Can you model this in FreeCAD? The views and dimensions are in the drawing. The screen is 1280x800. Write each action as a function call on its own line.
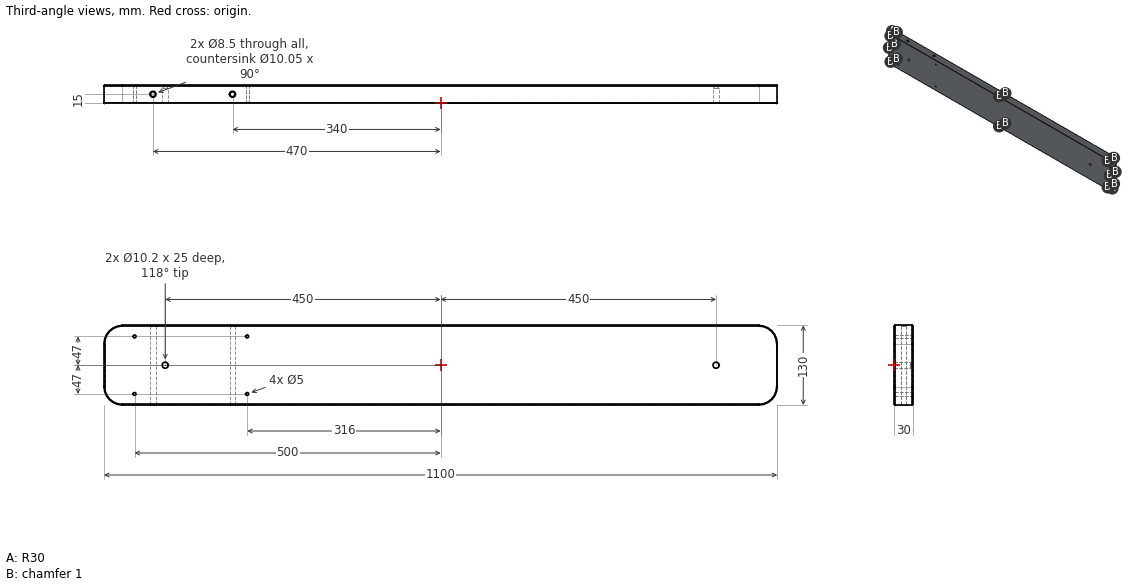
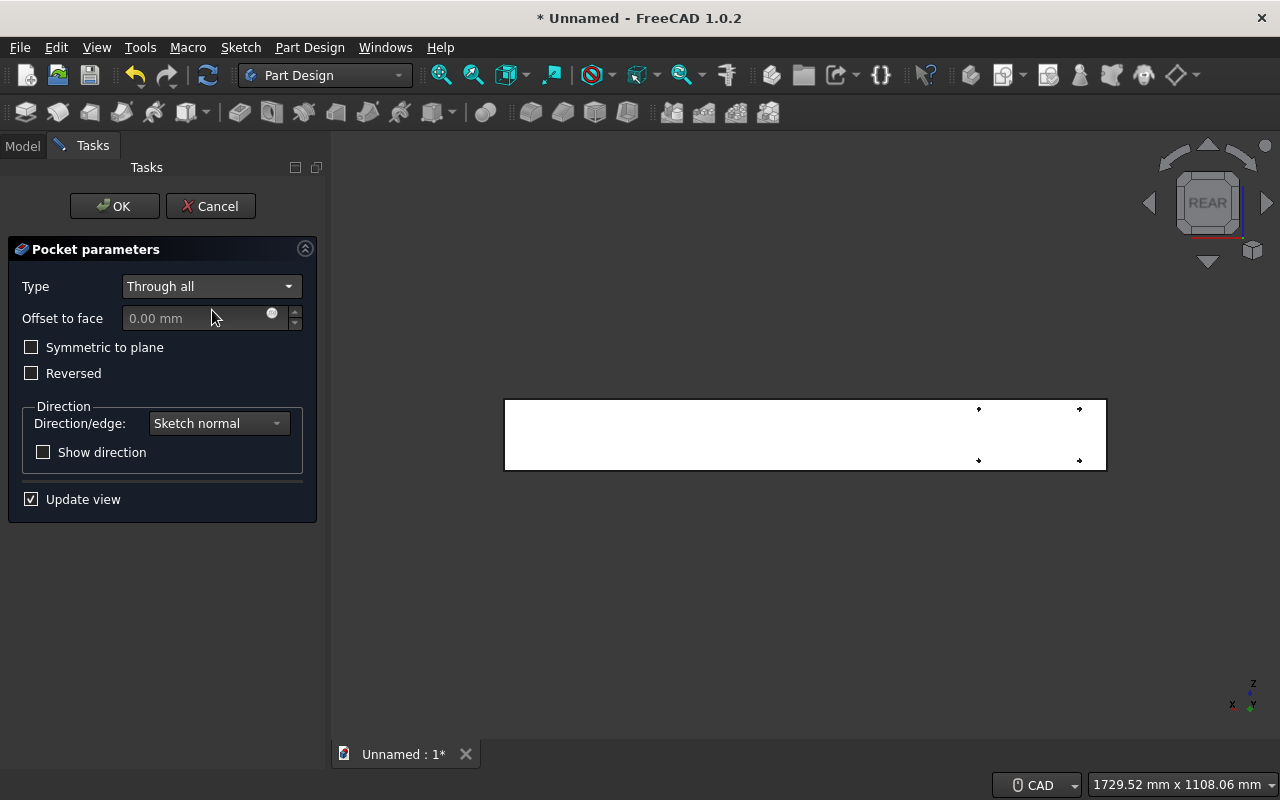
click(115, 206)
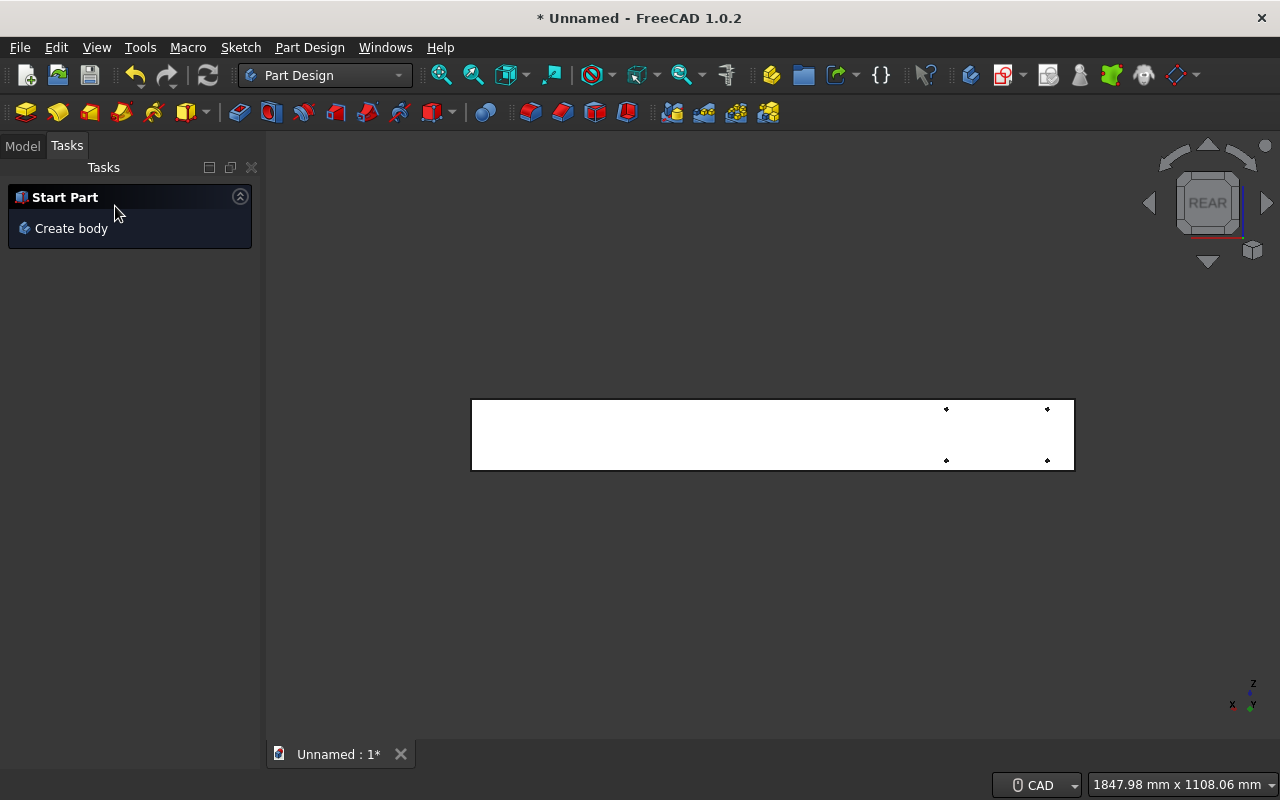
key(0)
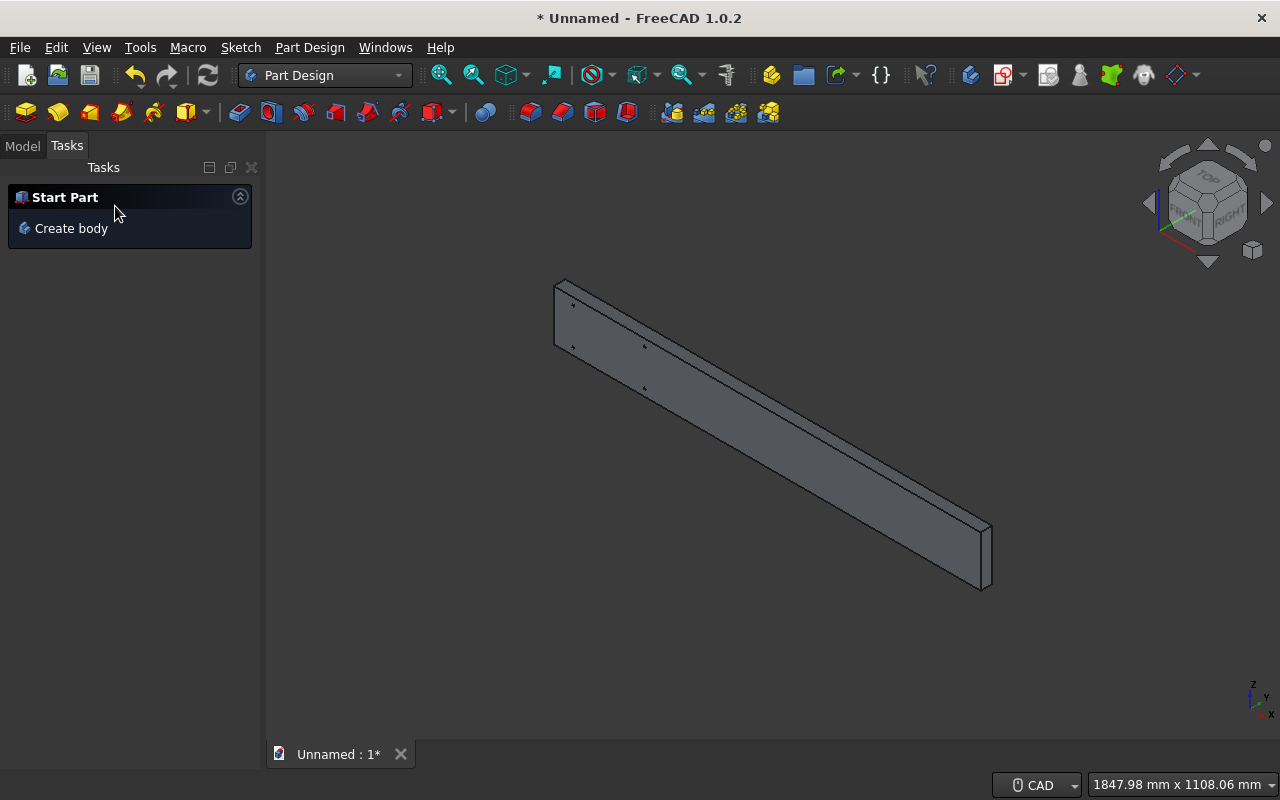
click(950, 543)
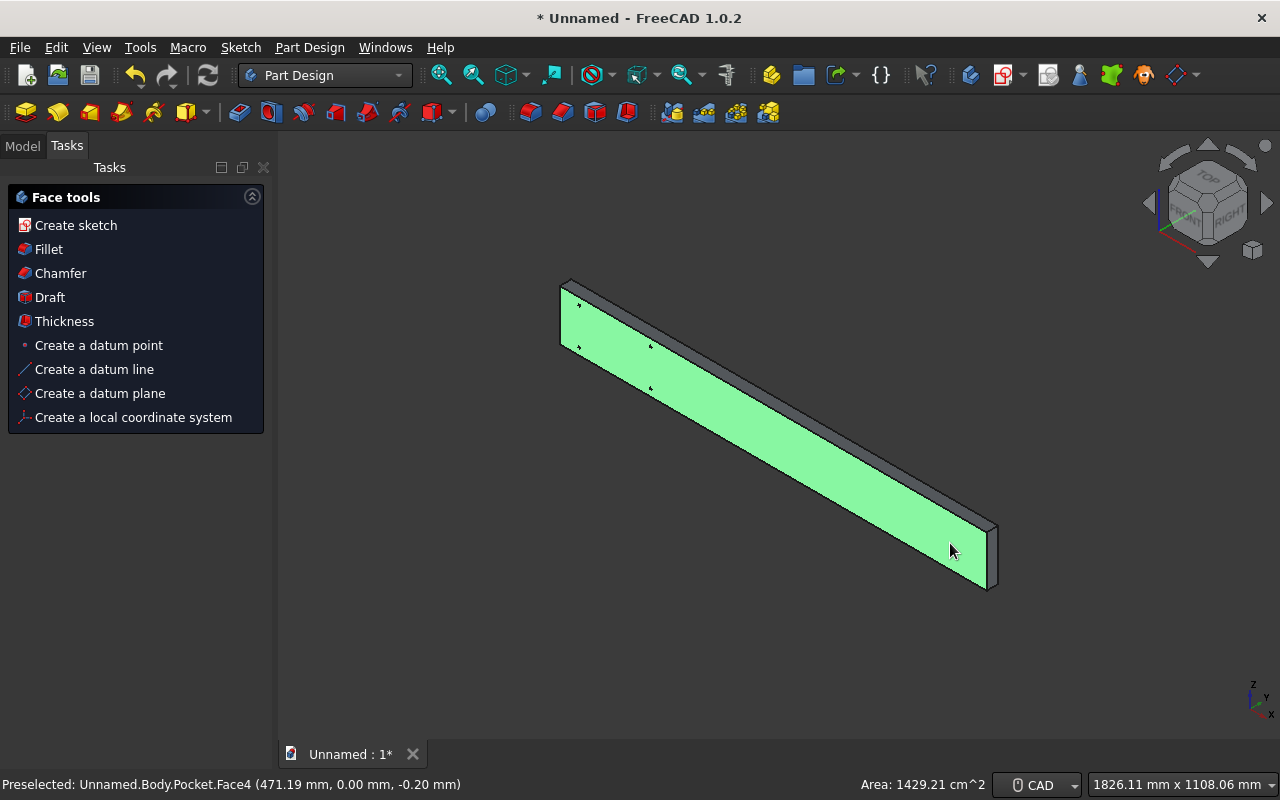
click(1004, 76)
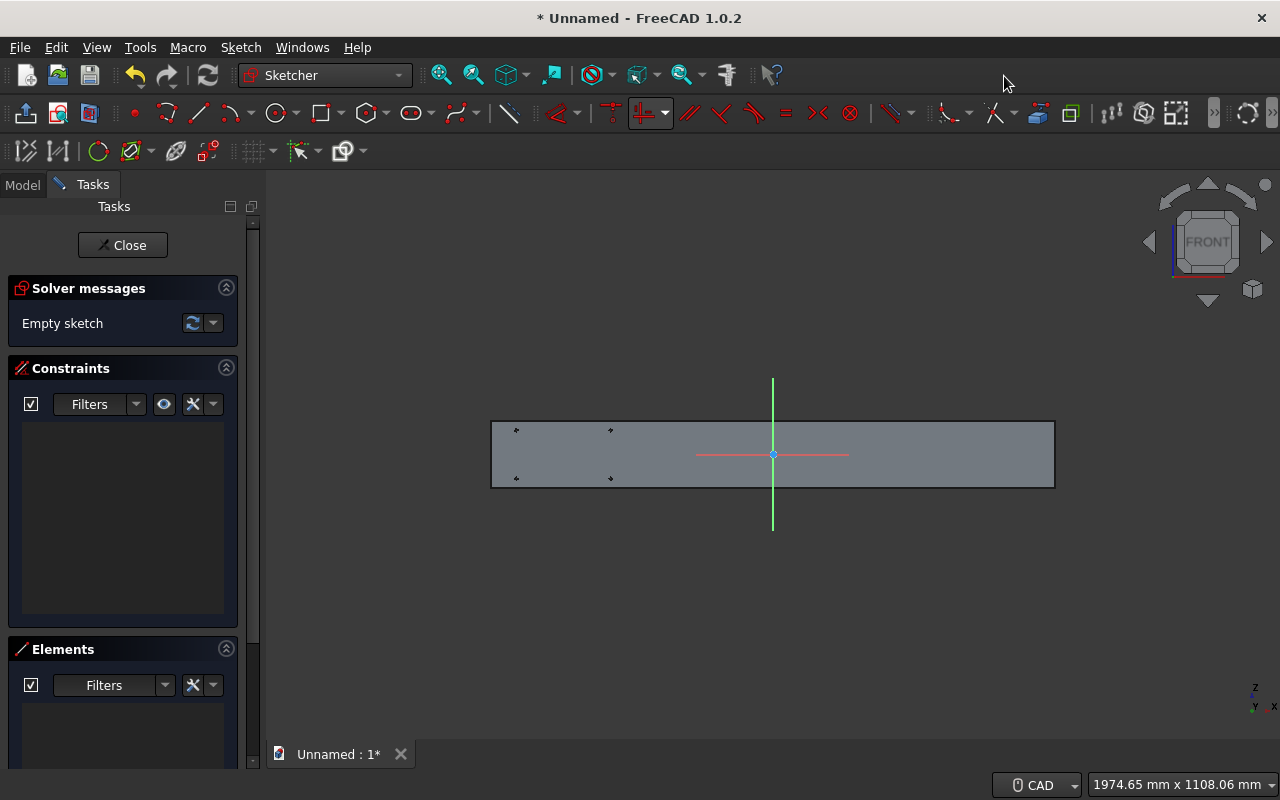
click(276, 114)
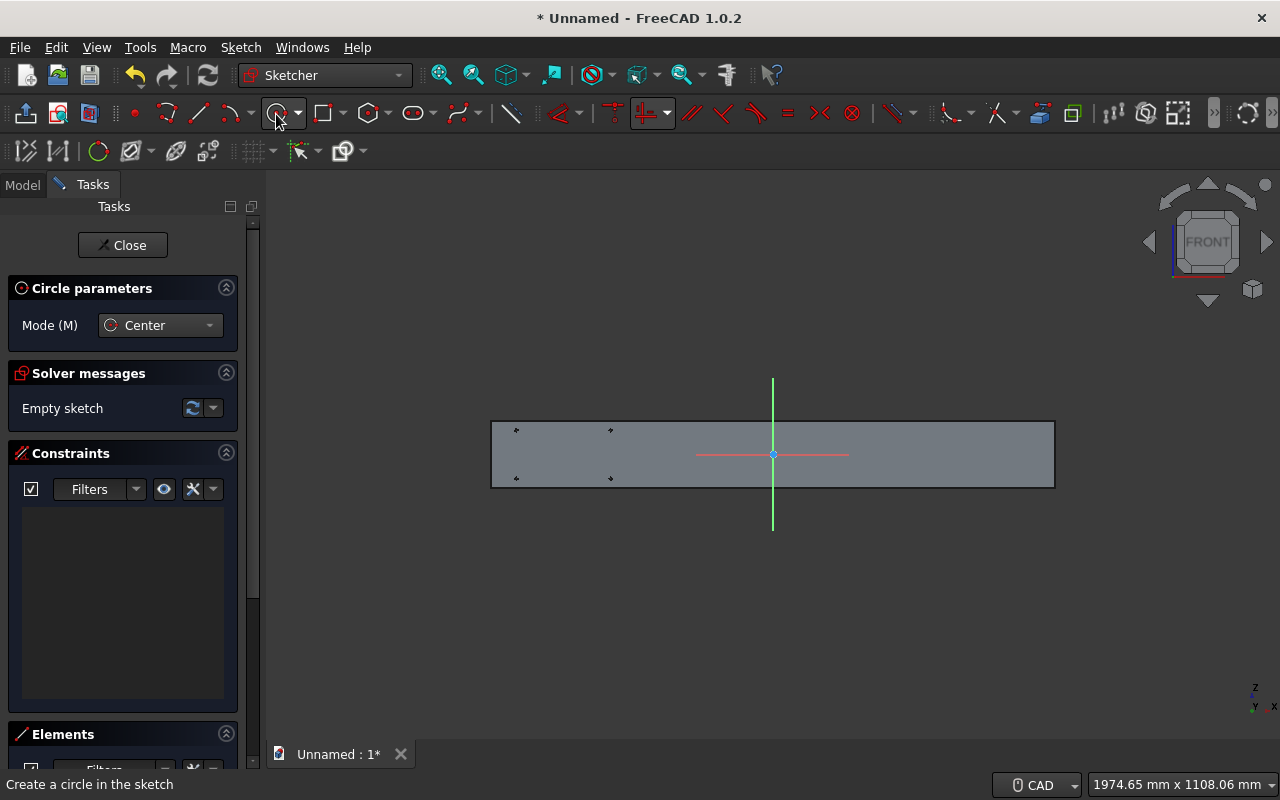
scroll(542, 455, up, 11)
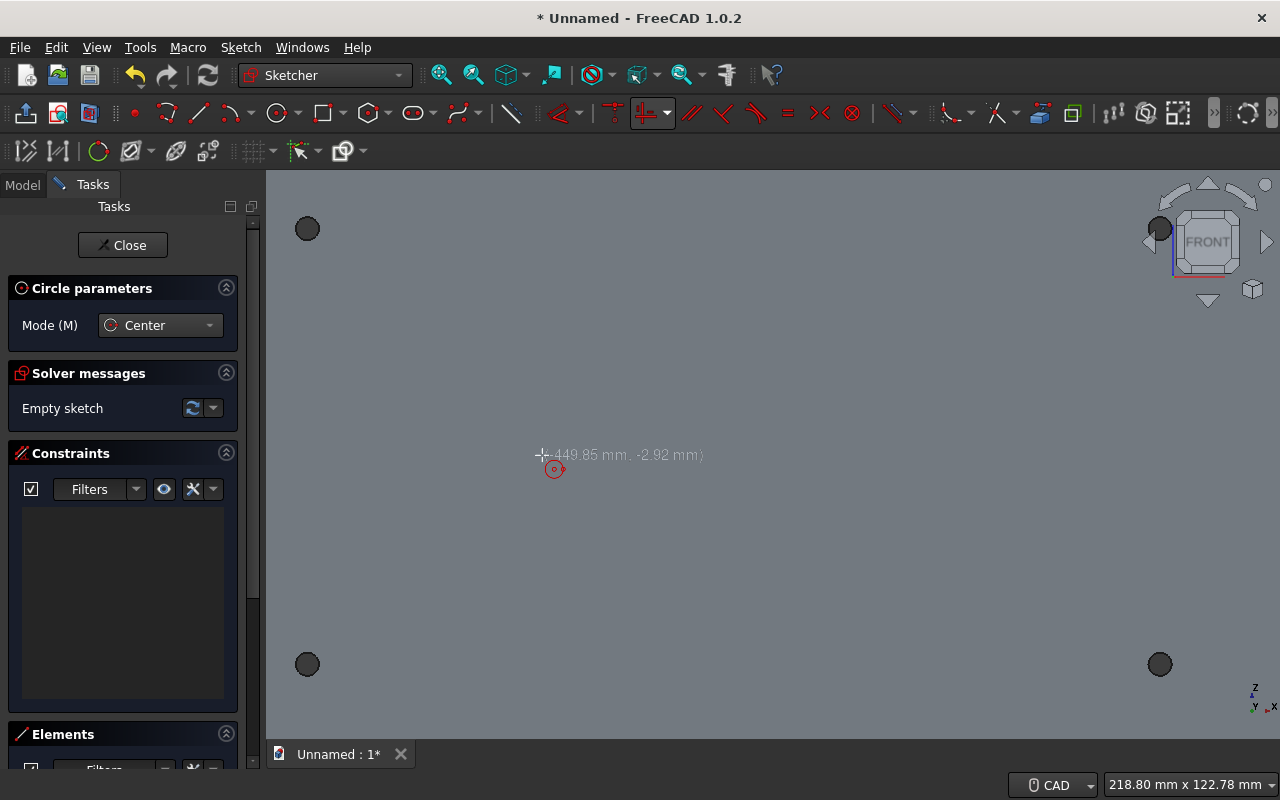
scroll(404, 456, down, 10)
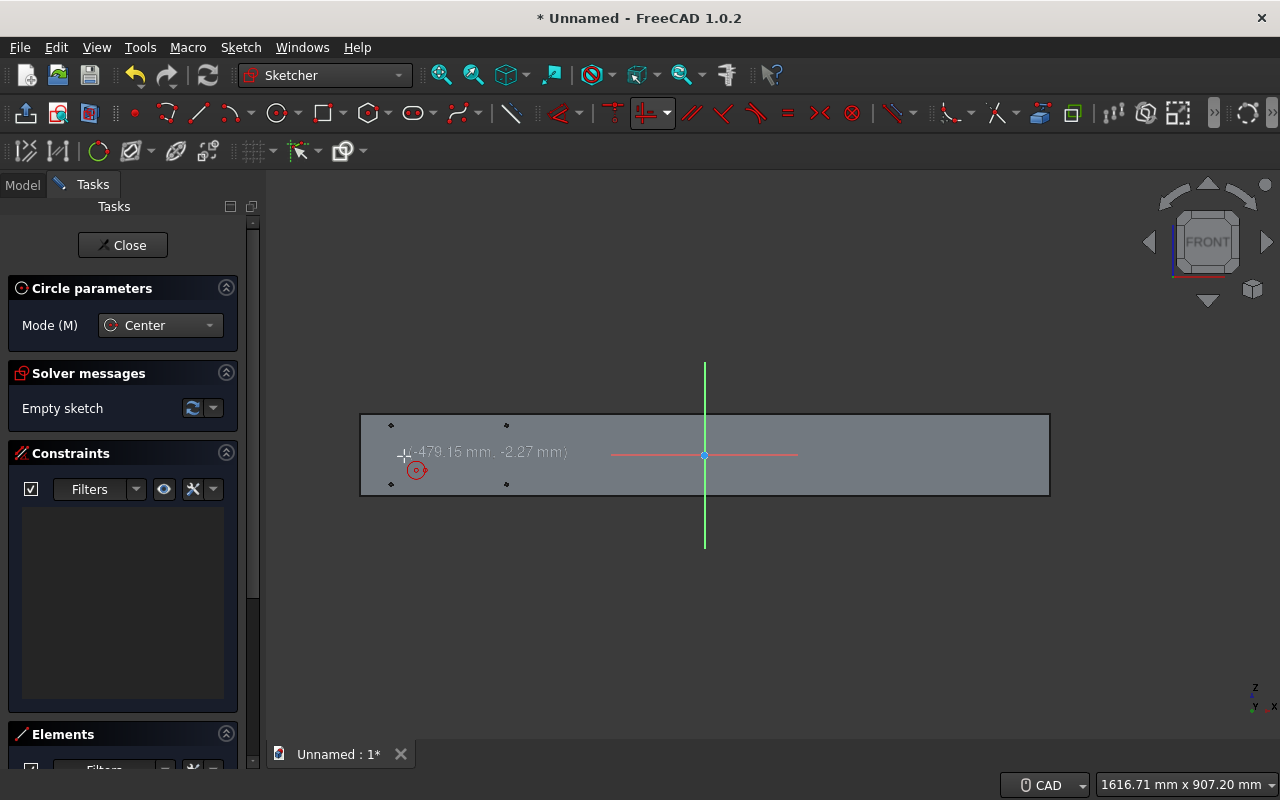
click(422, 455)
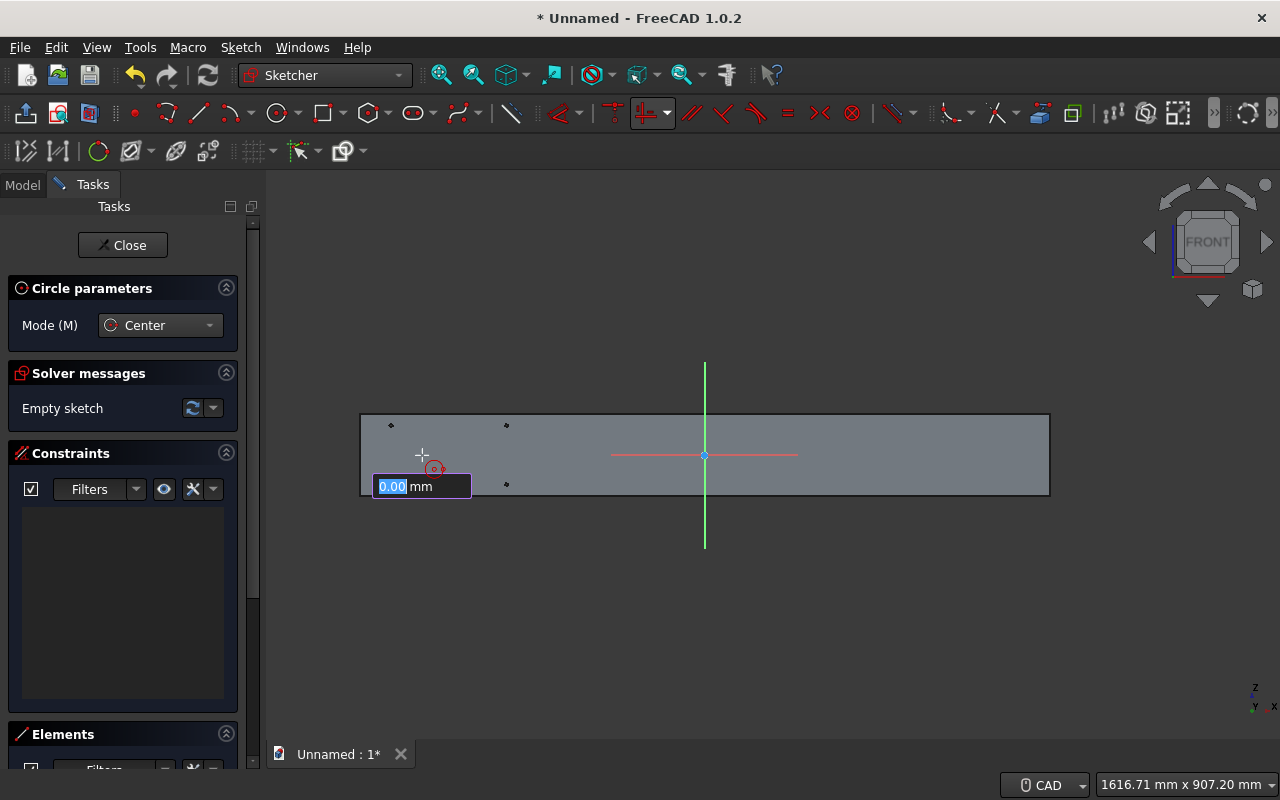
scroll(421, 458, up, 9)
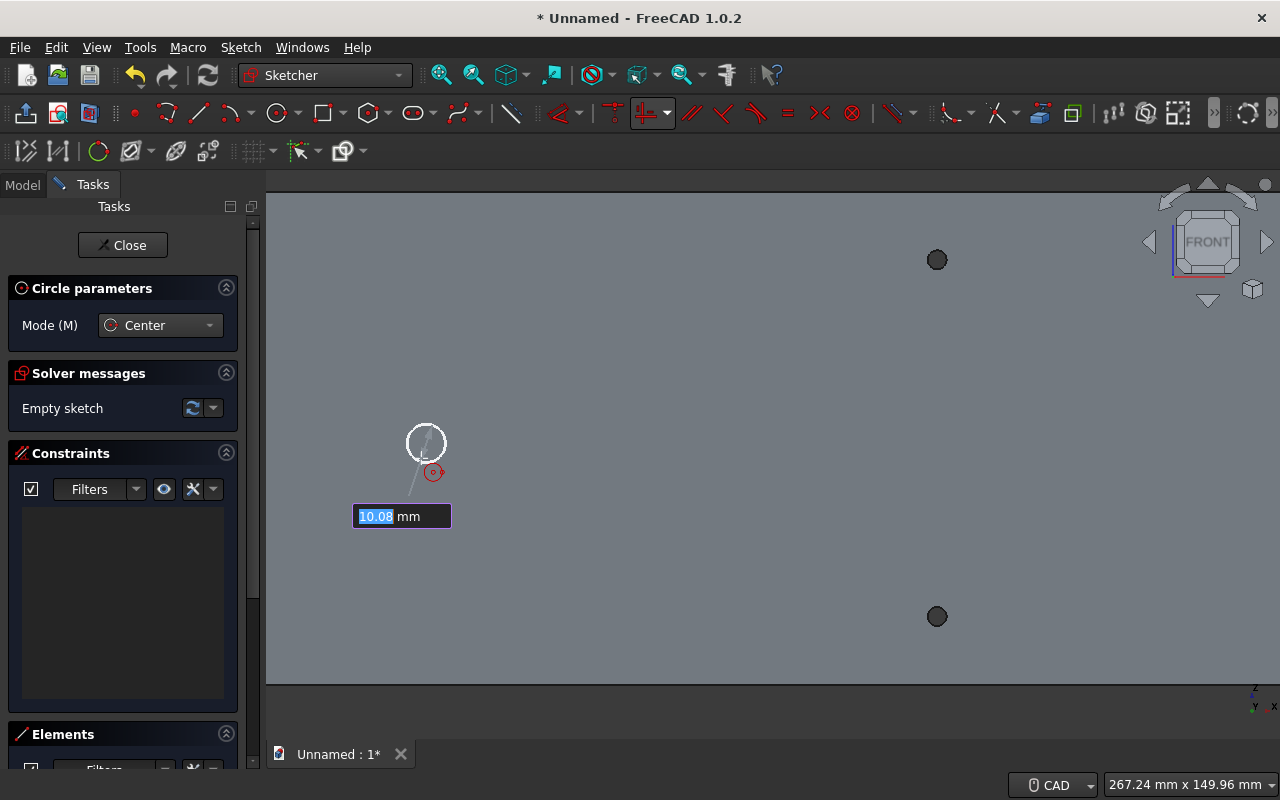
click(422, 456)